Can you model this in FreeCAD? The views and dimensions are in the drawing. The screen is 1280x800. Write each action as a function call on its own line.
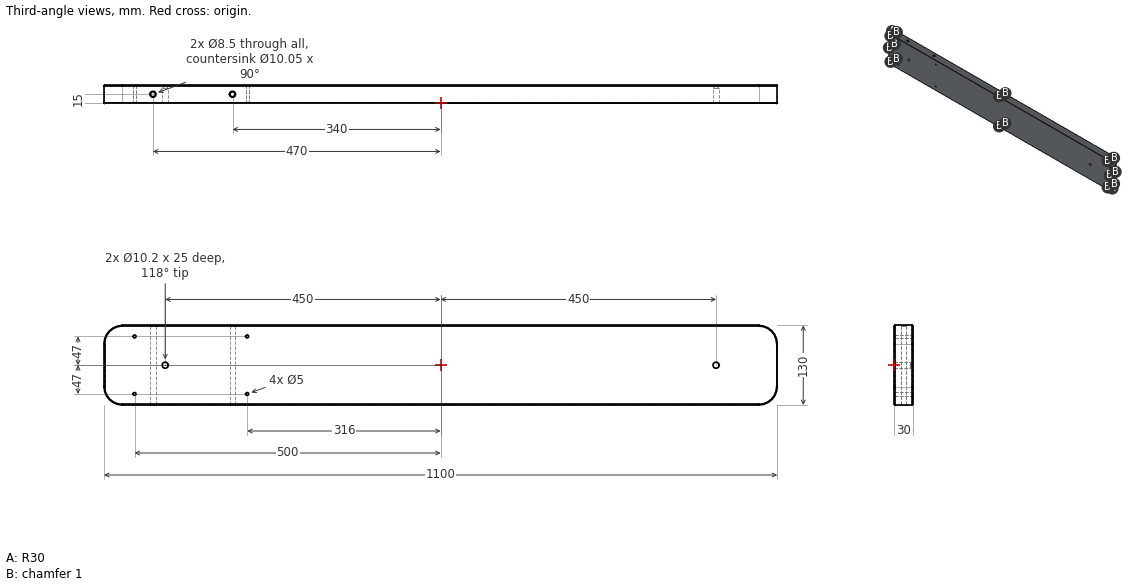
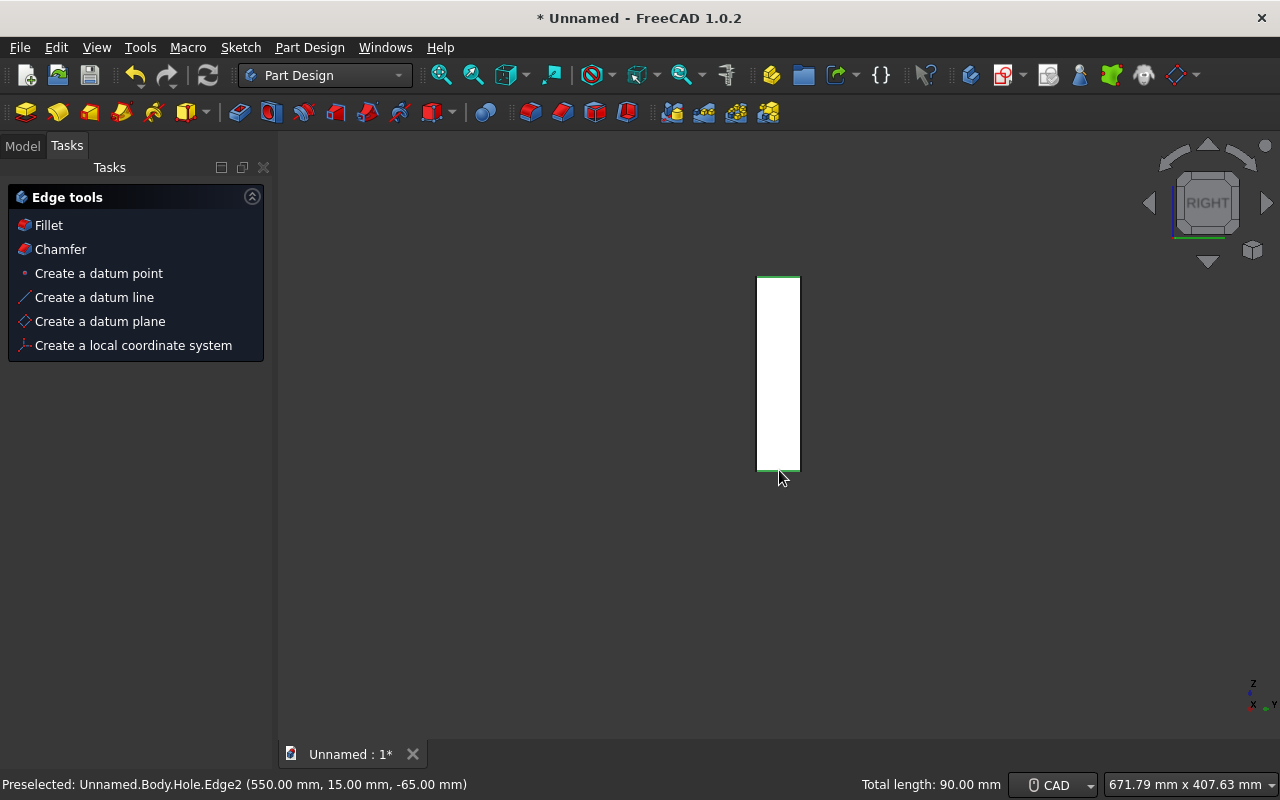
click(442, 76)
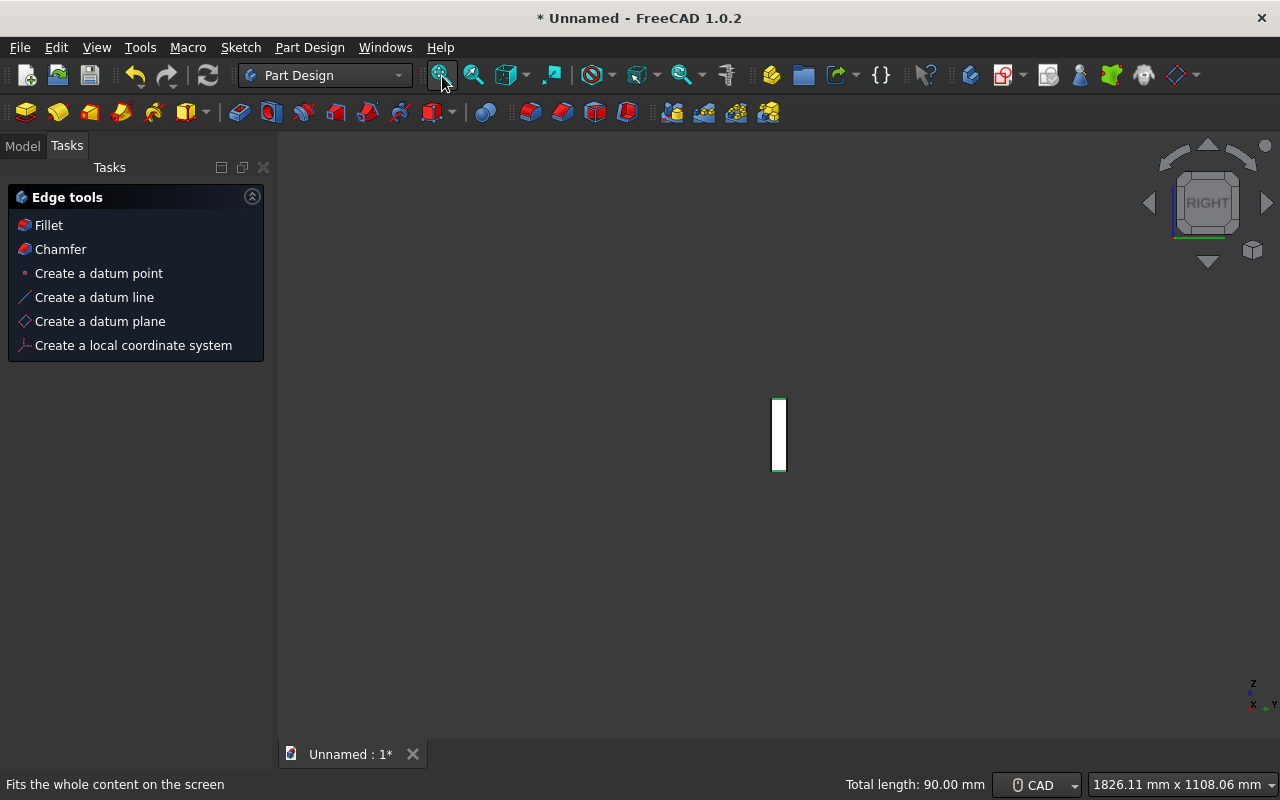
key(5)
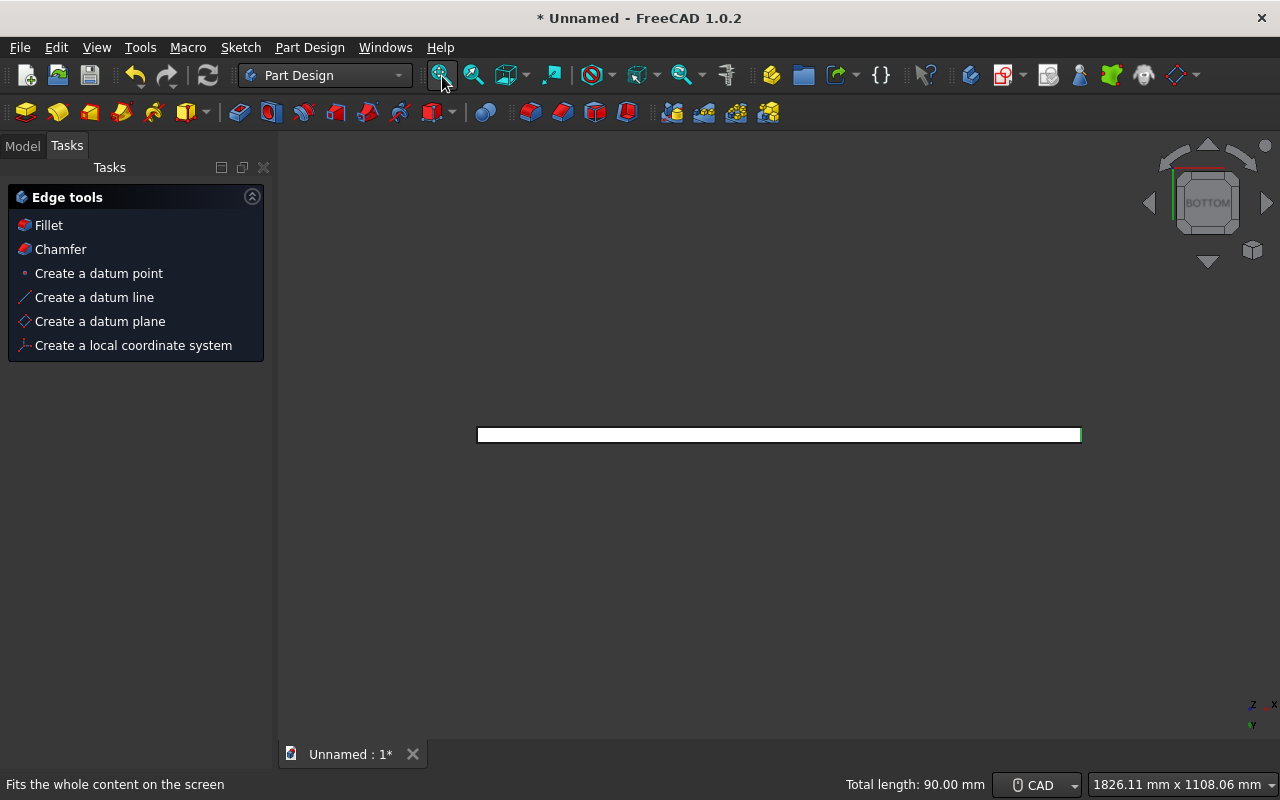
click(477, 434, ctrl)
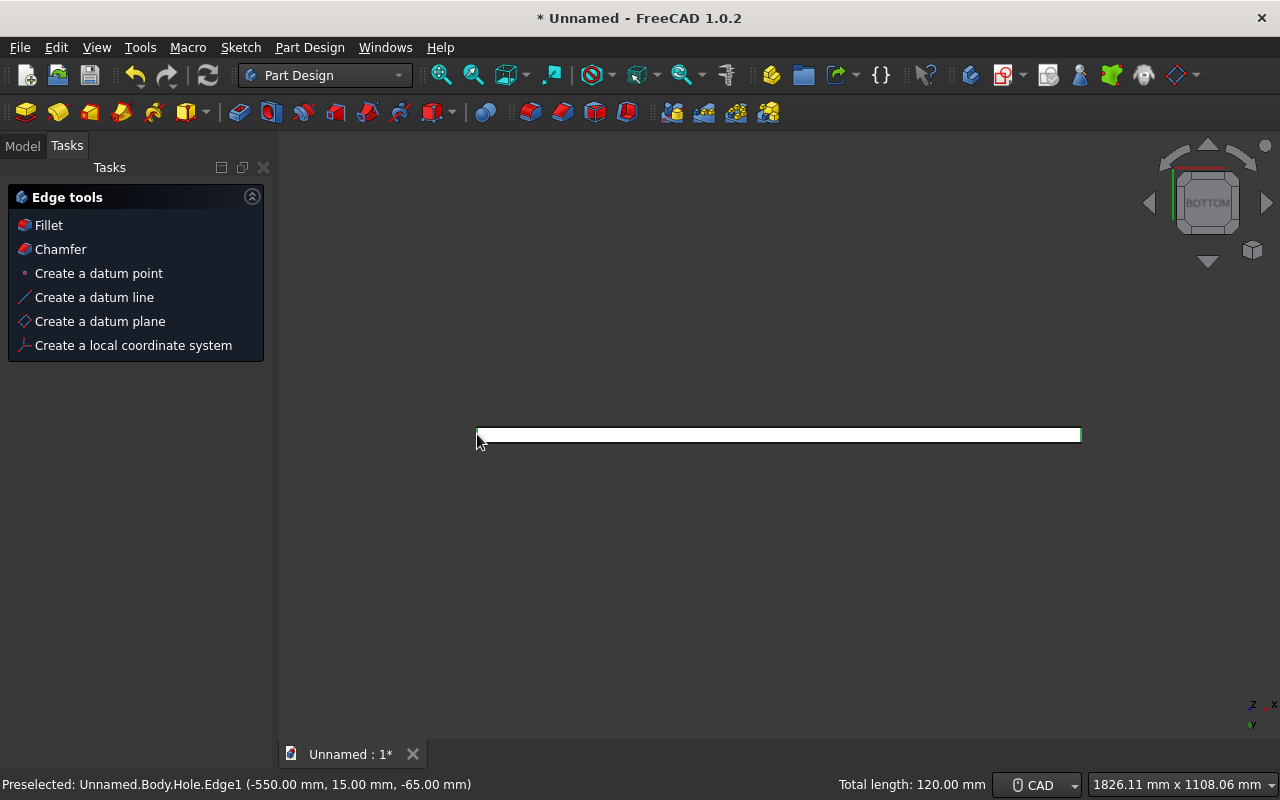
click(532, 112)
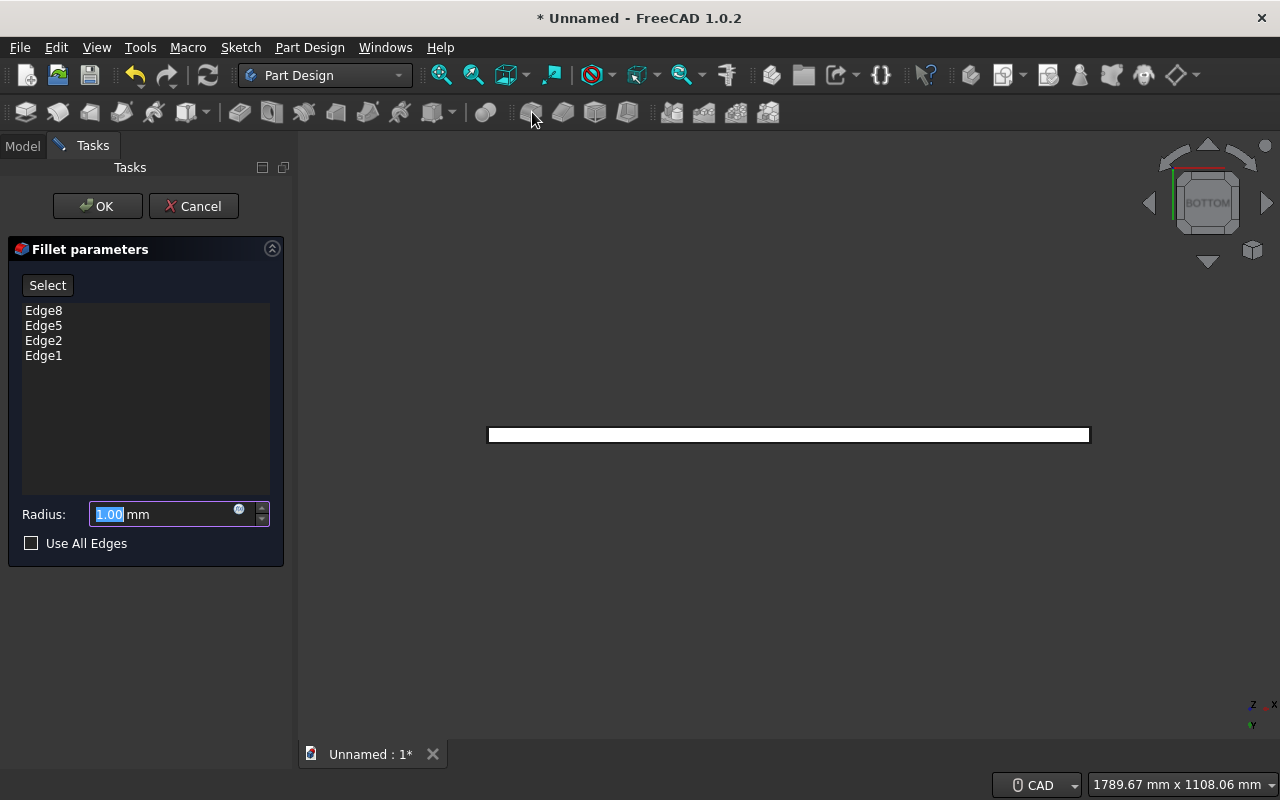
text(30)
key(Tab)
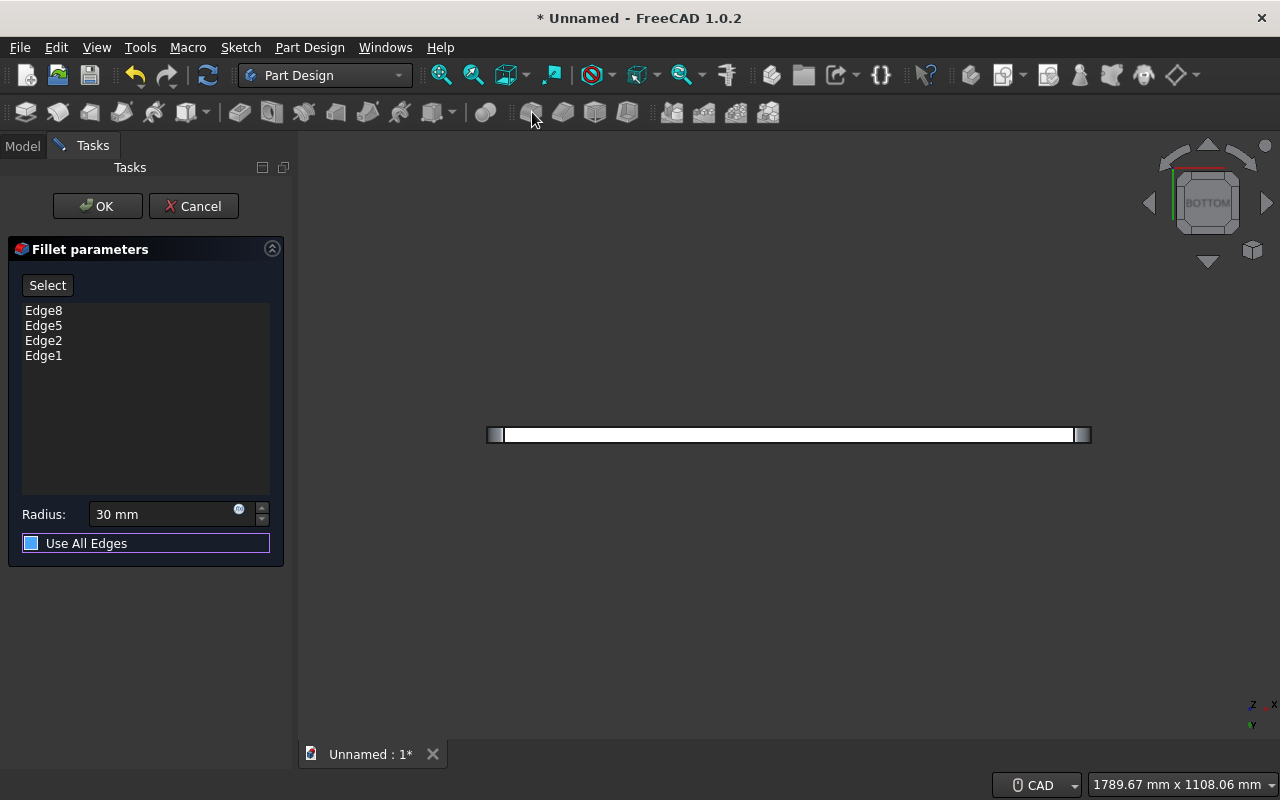
click(98, 206)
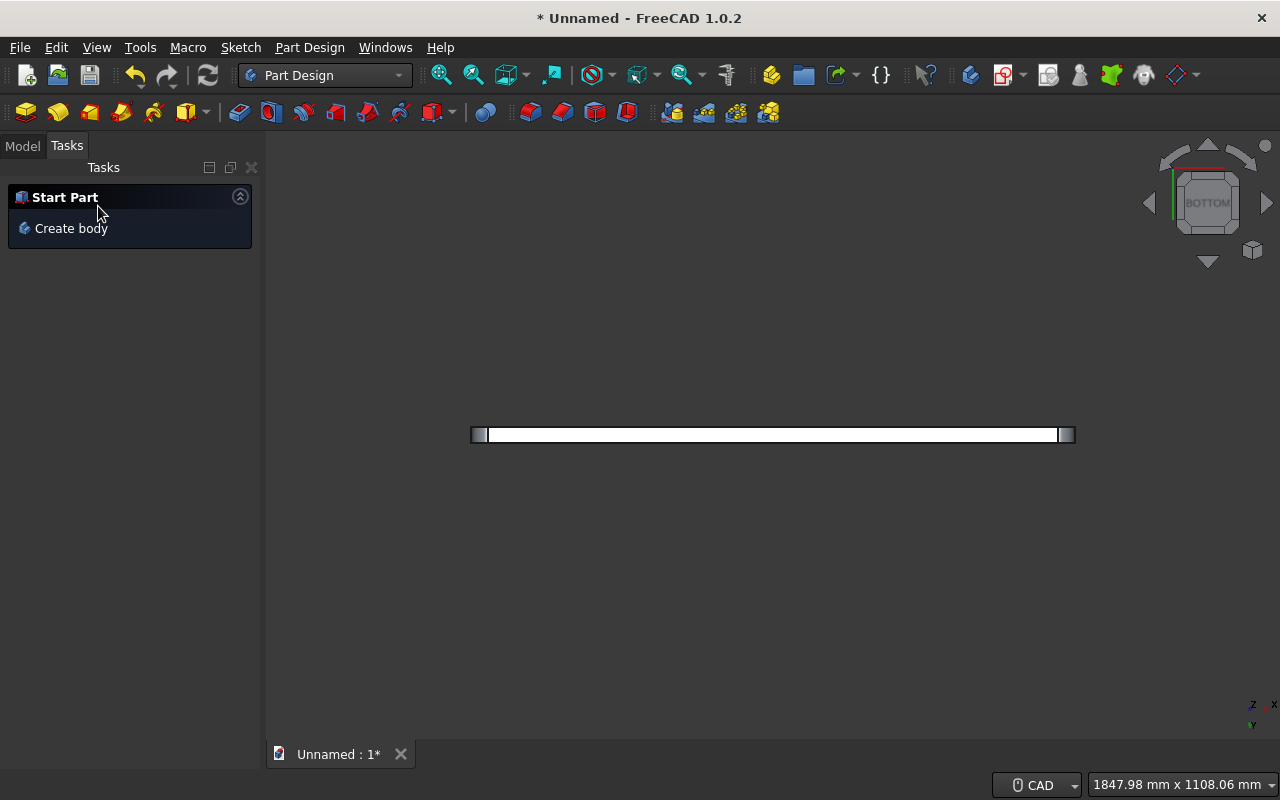
click(773, 426)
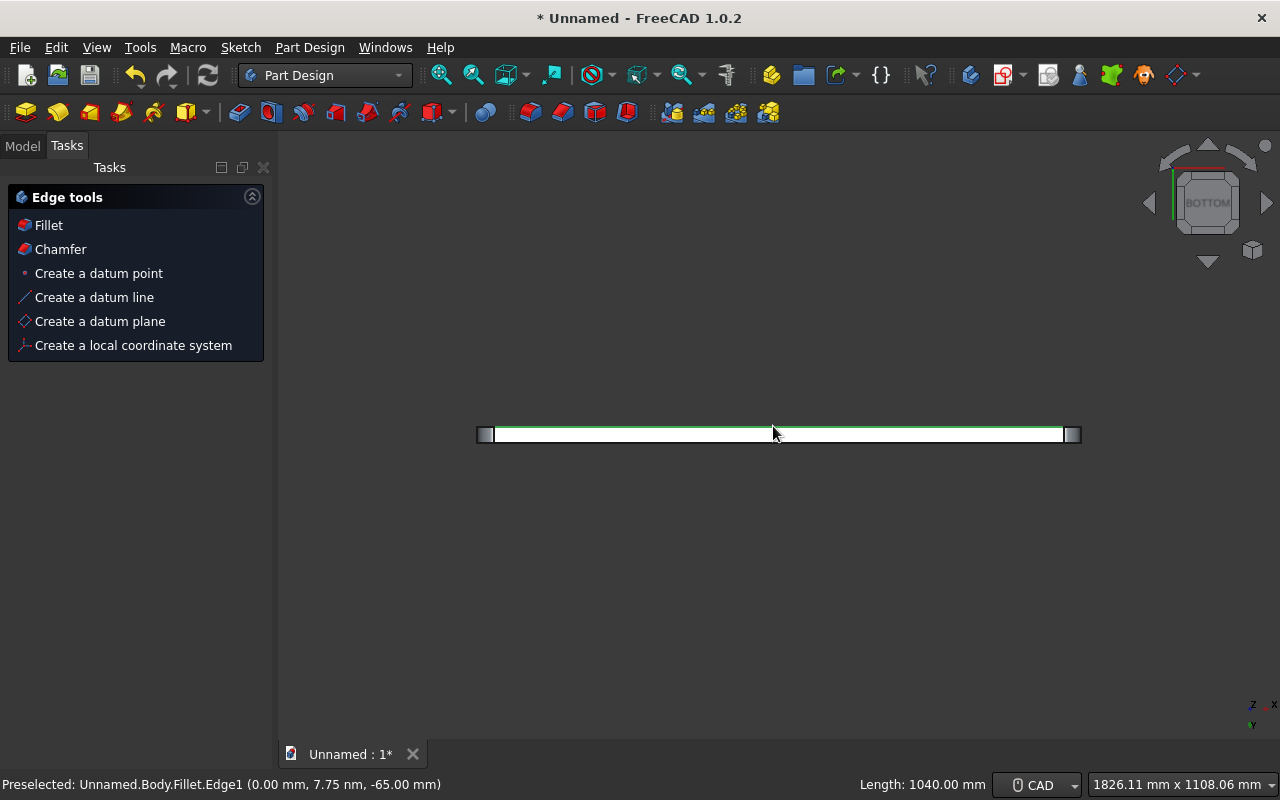
click(1076, 426, ctrl)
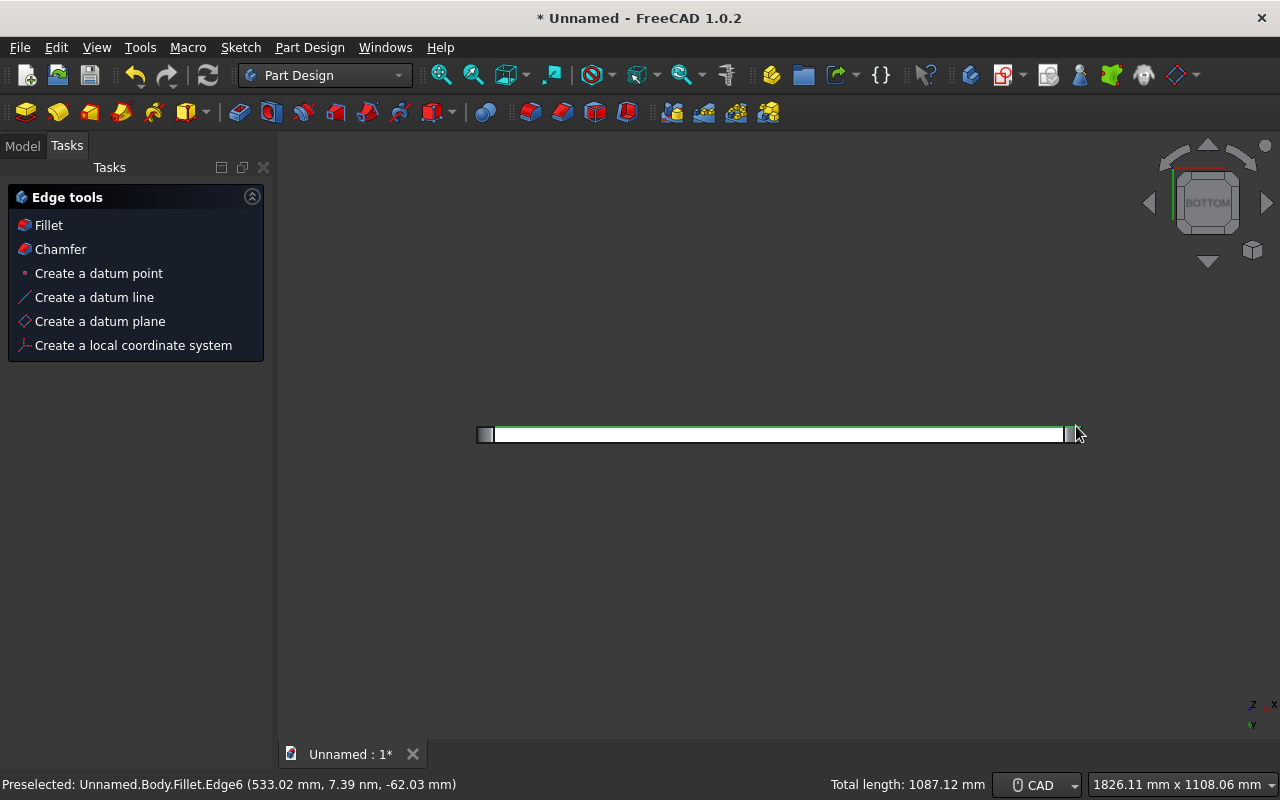
click(482, 426, ctrl)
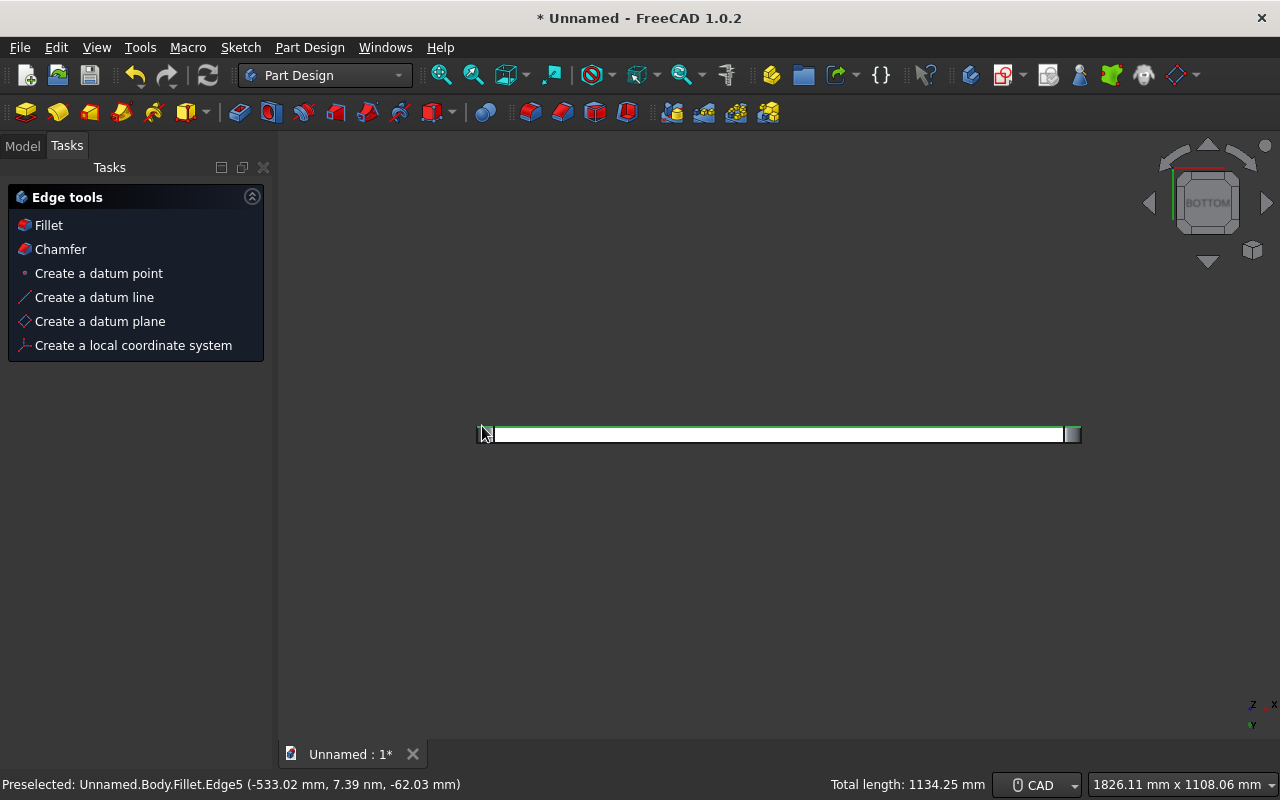
click(1076, 442, ctrl)